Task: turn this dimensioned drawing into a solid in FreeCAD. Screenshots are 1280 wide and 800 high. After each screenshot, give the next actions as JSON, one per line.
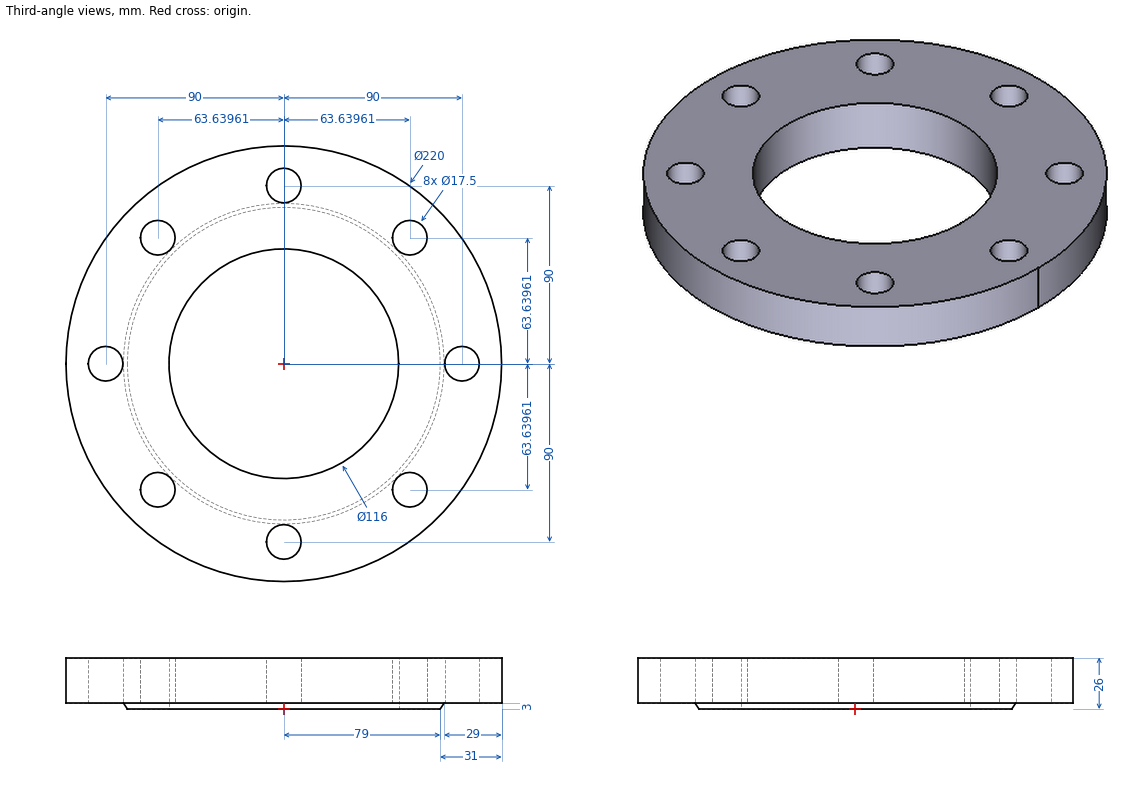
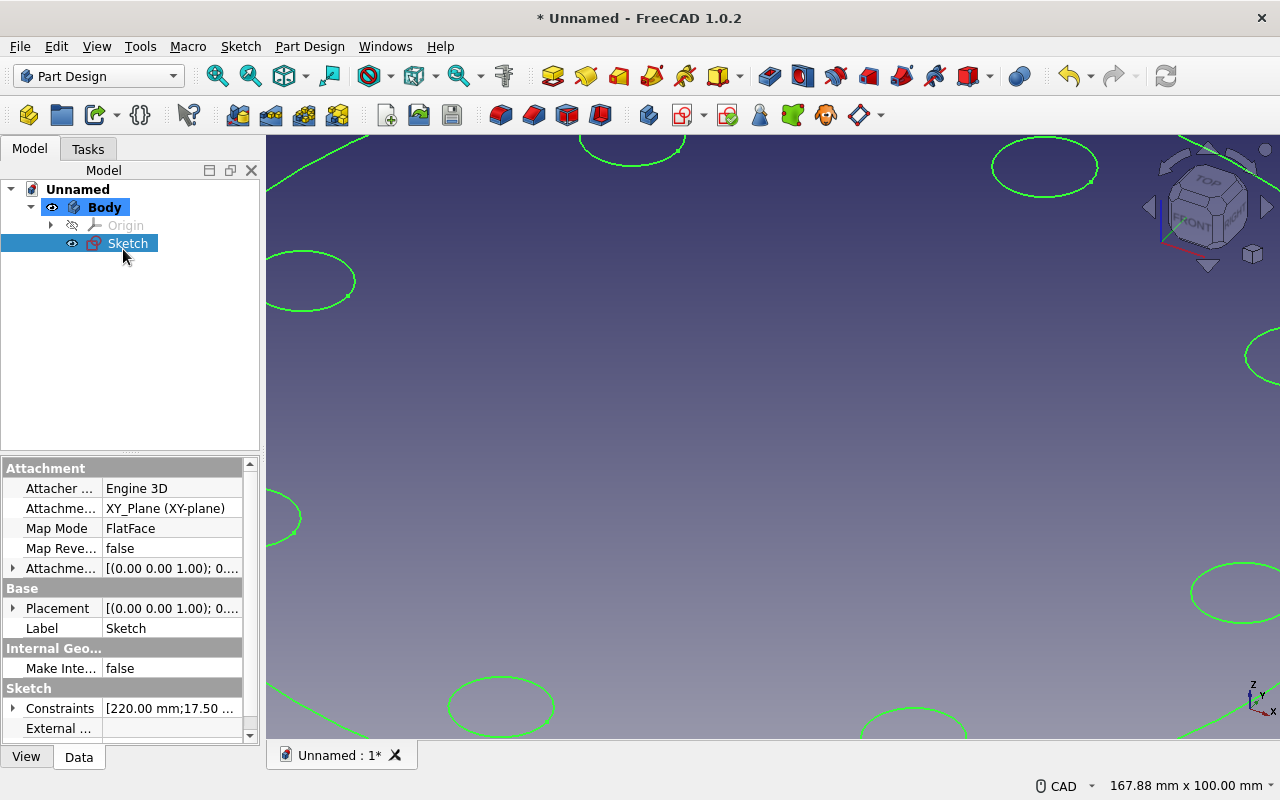
{"action": "left_click", "coordinate": [553, 76]}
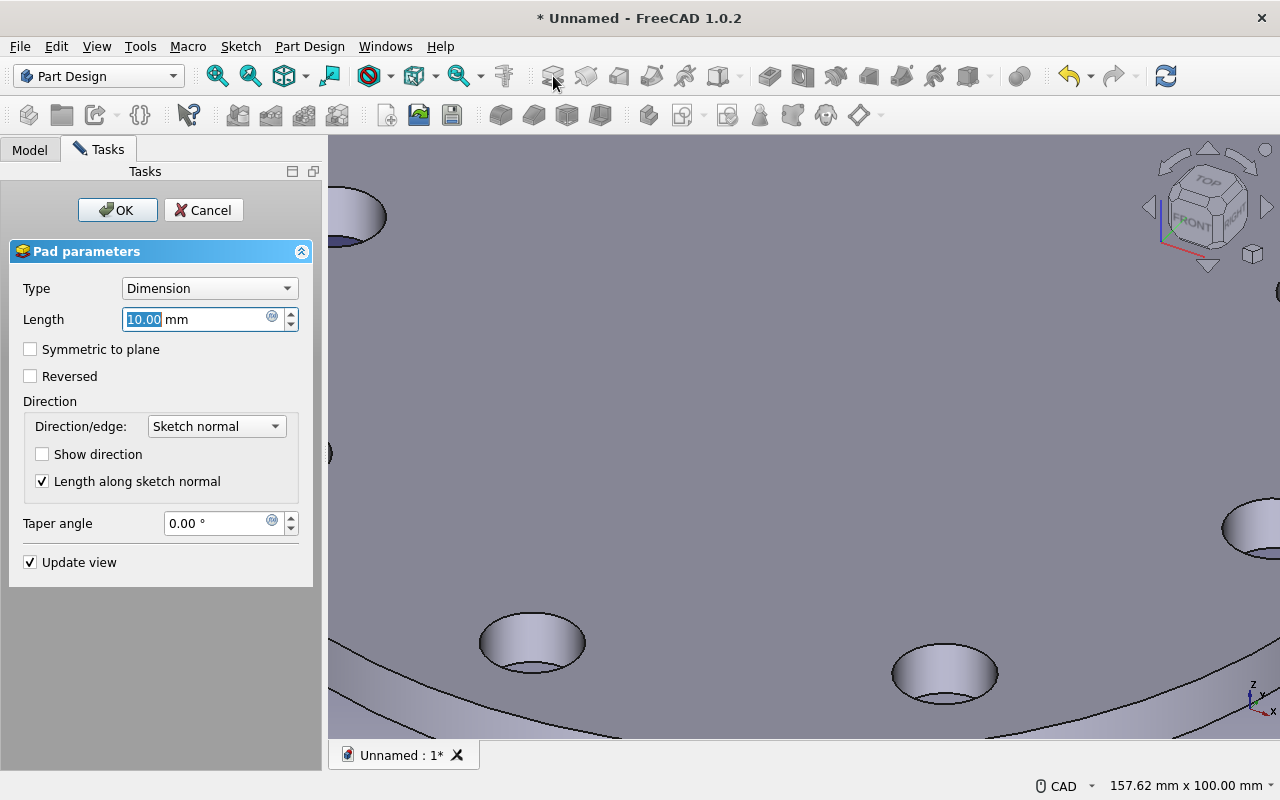
{"action": "type", "text": "26"}
{"action": "key", "text": "Tab"}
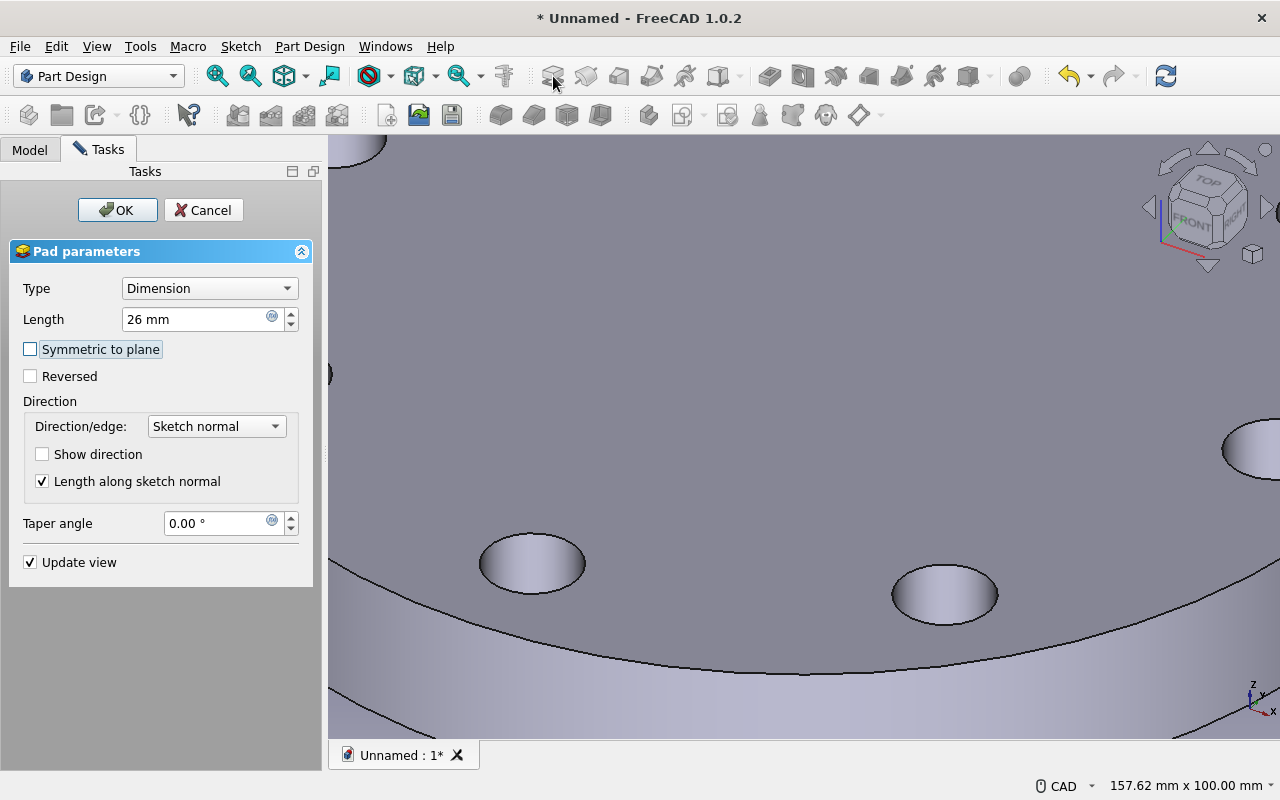
{"action": "left_click", "coordinate": [118, 210]}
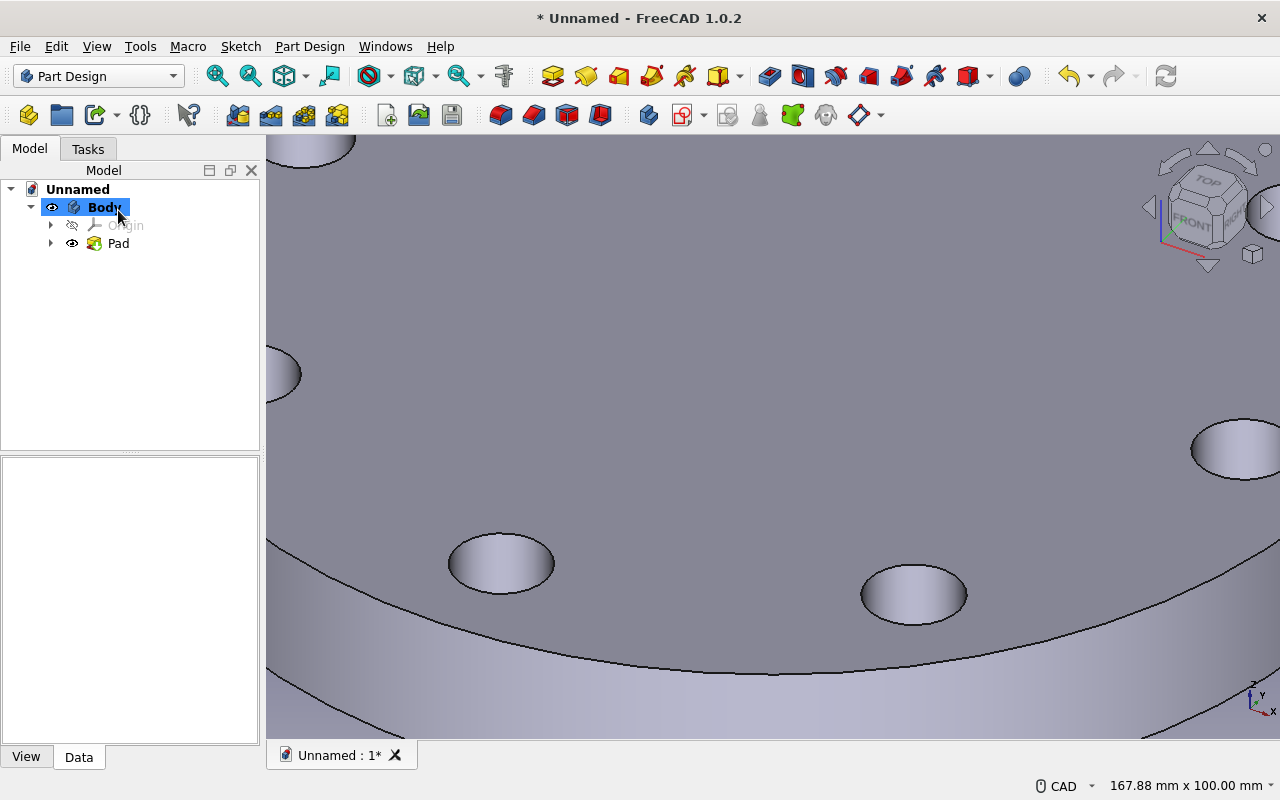
{"action": "left_click", "coordinate": [218, 76]}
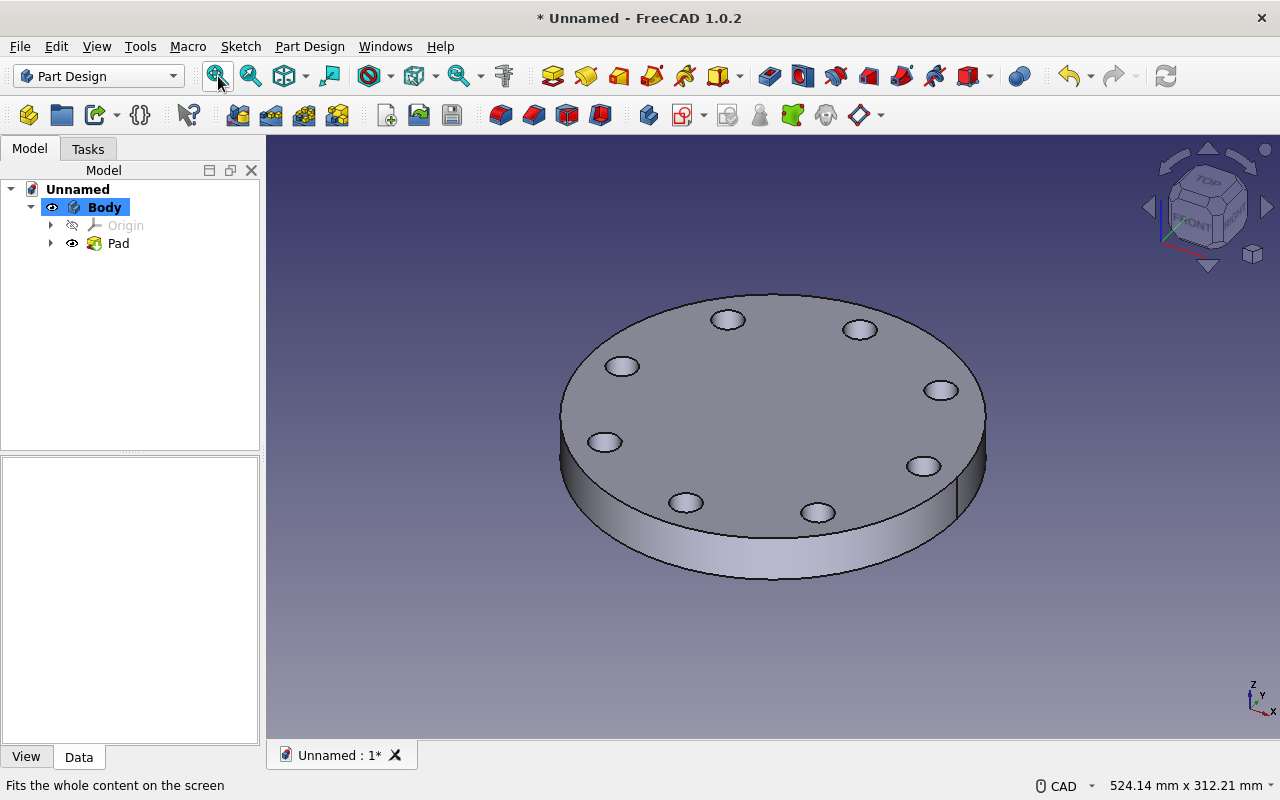
{"action": "left_click", "coordinate": [773, 415]}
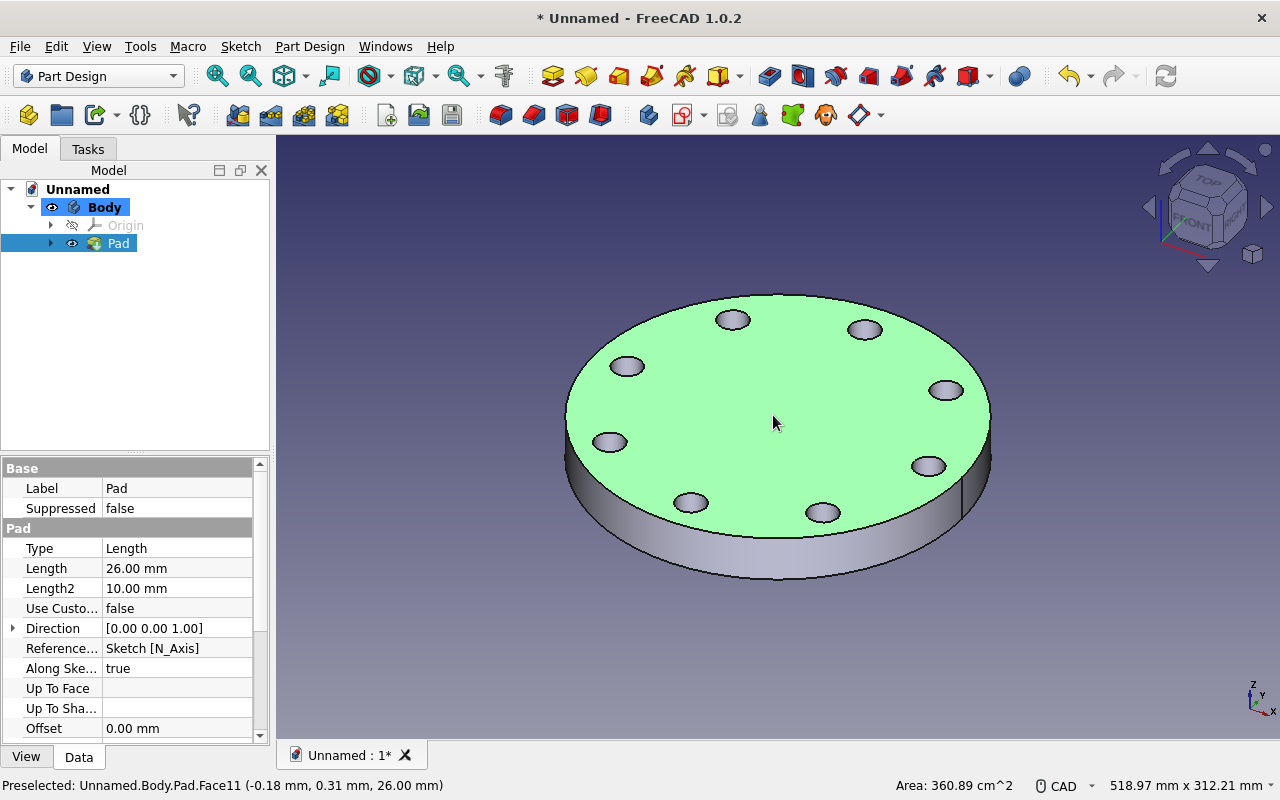
{"action": "left_click", "coordinate": [682, 116]}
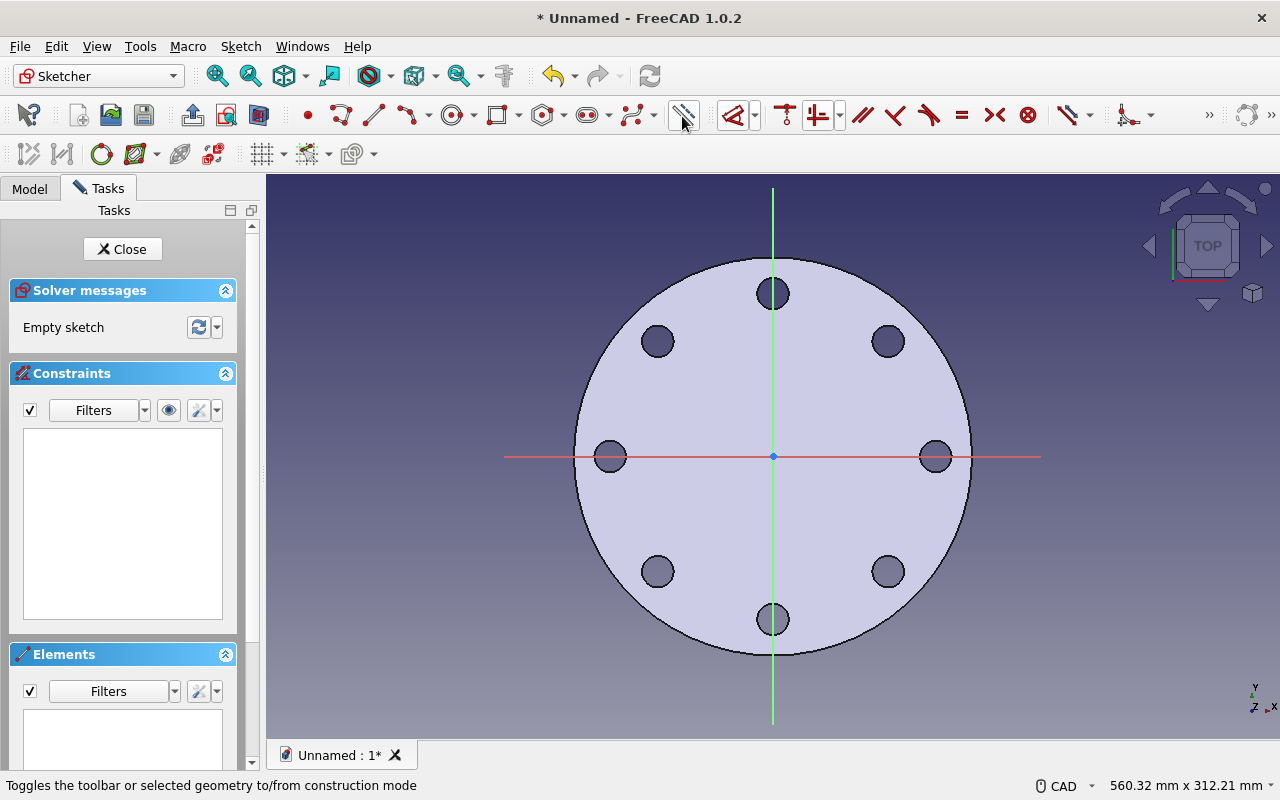
{"action": "scroll", "coordinate": [856, 456], "scroll_direction": "up", "scroll_amount": 3}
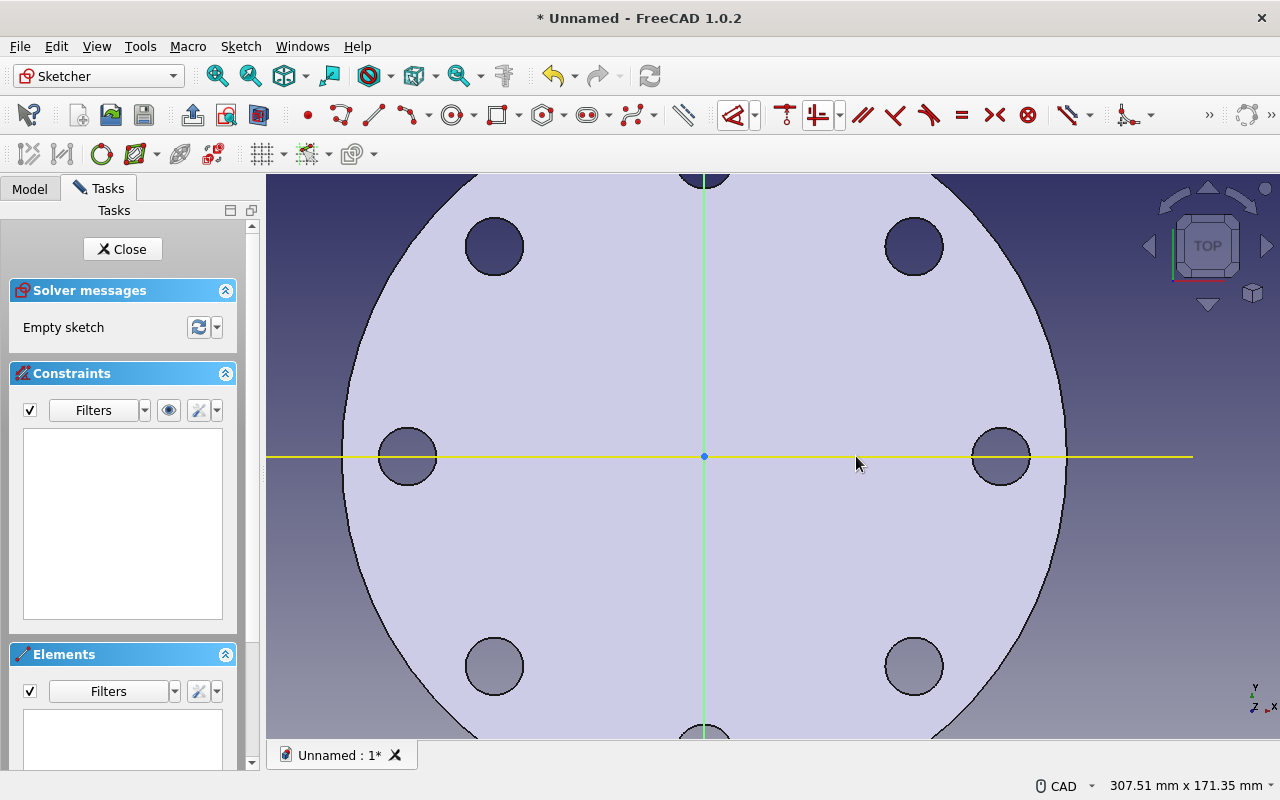
{"action": "left_click", "coordinate": [452, 116]}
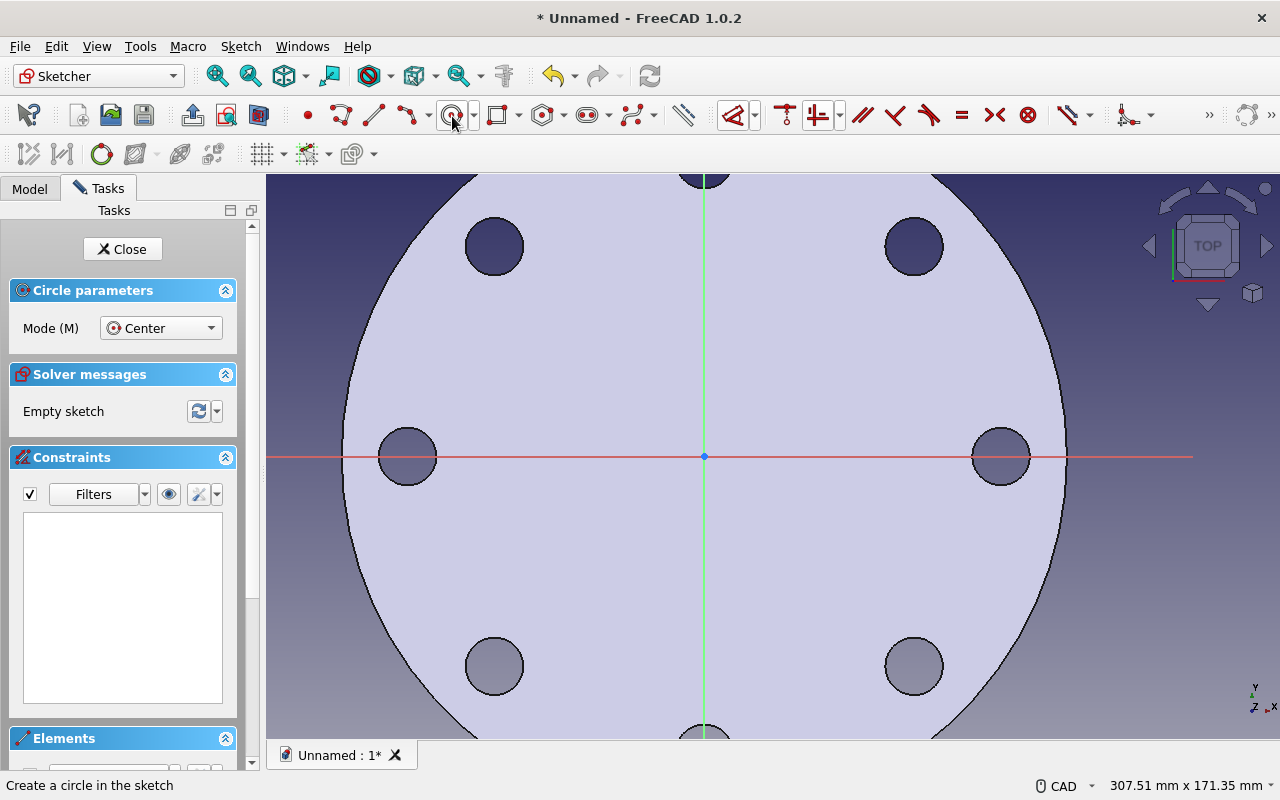
{"action": "left_click", "coordinate": [704, 456]}
{"action": "left_click", "coordinate": [840, 321]}
{"action": "key", "text": "Escape"}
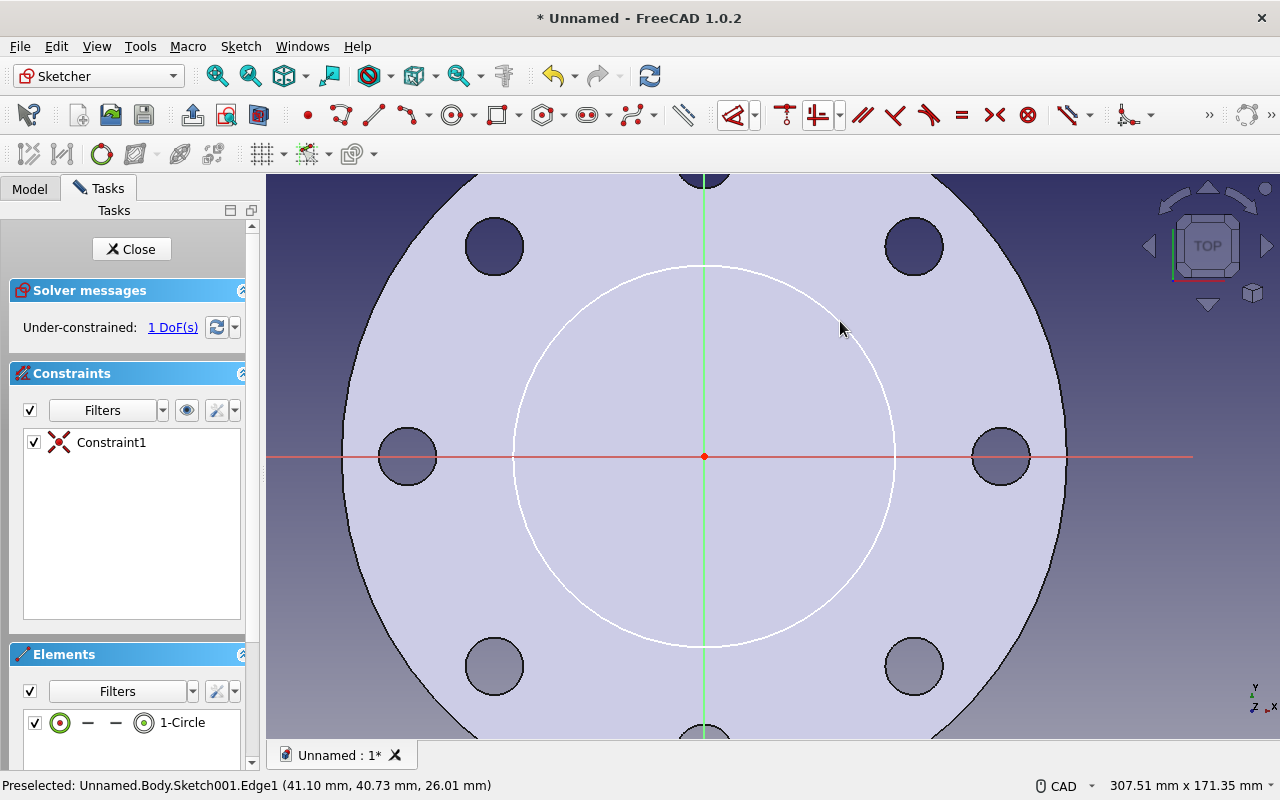
{"action": "left_click", "coordinate": [839, 321]}